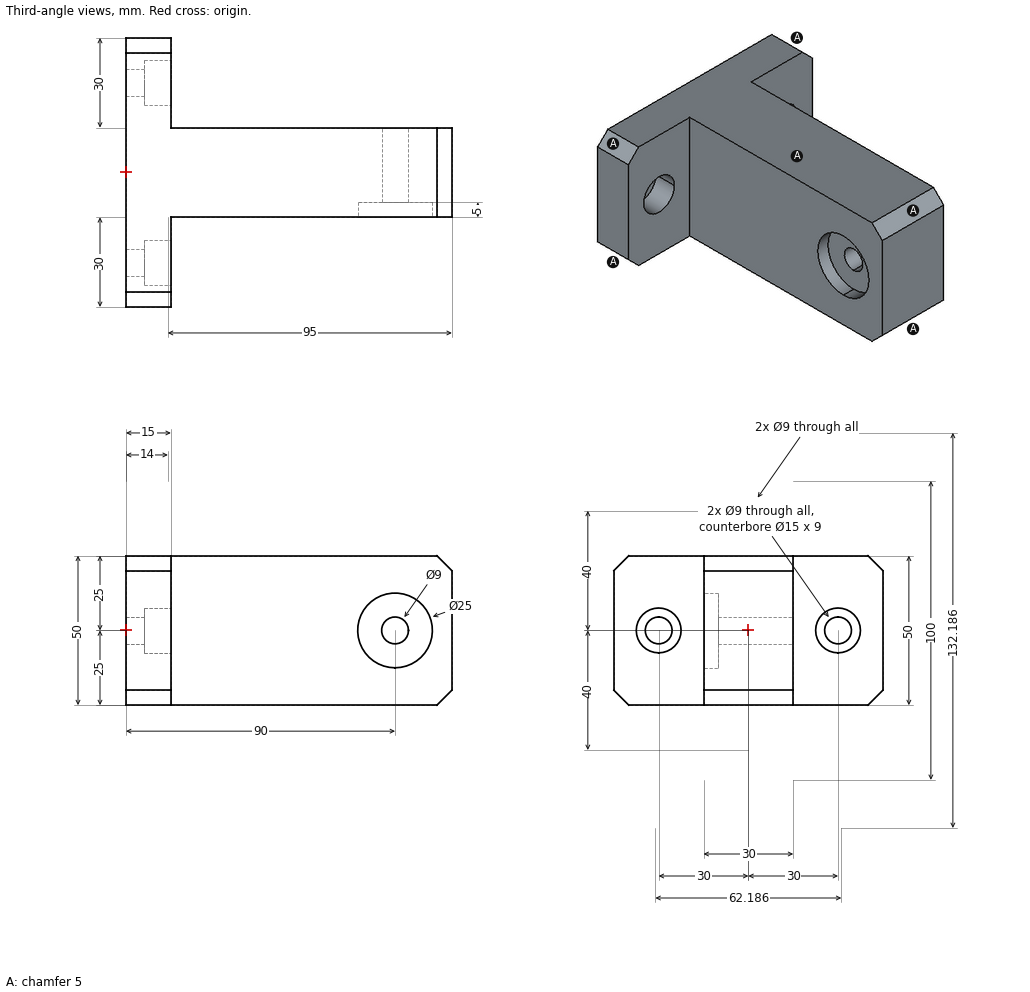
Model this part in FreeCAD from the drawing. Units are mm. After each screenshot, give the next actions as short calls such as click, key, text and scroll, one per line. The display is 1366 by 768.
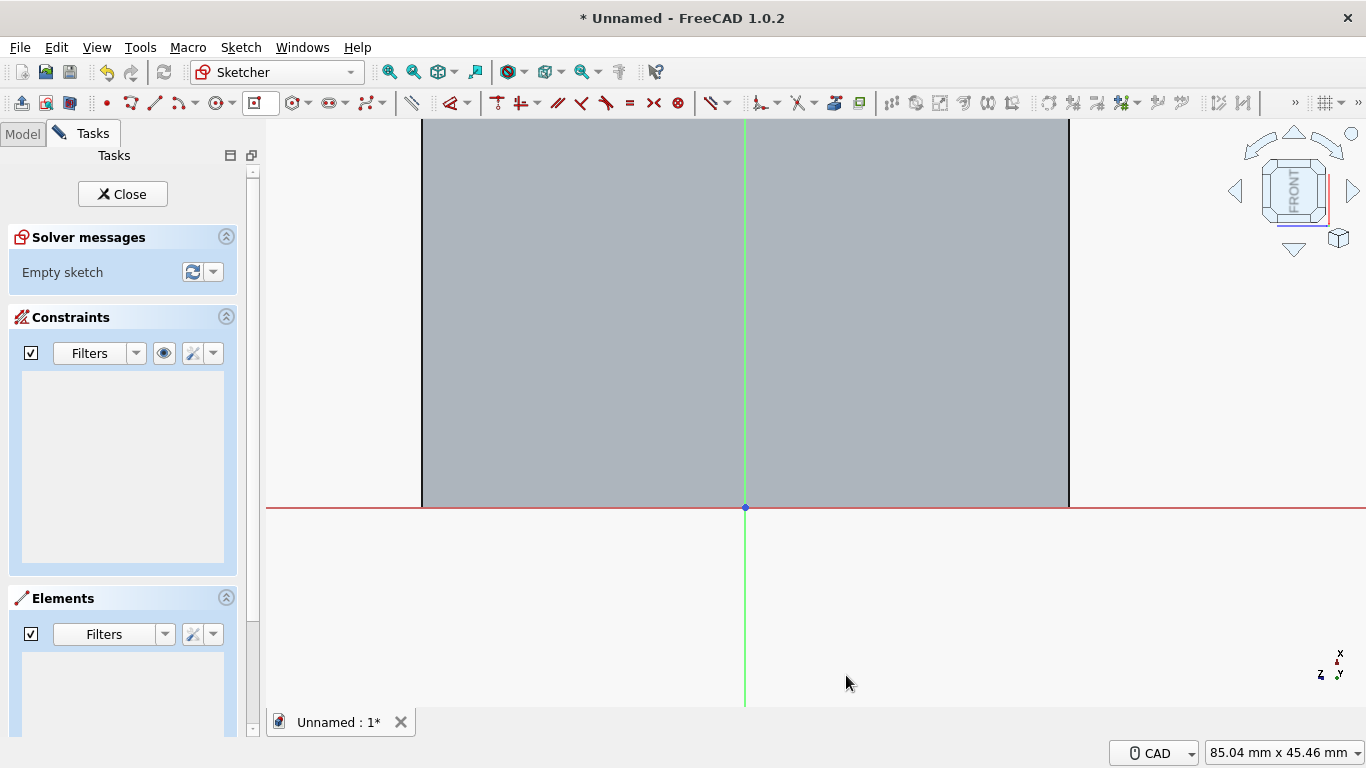
key(g)
key(r)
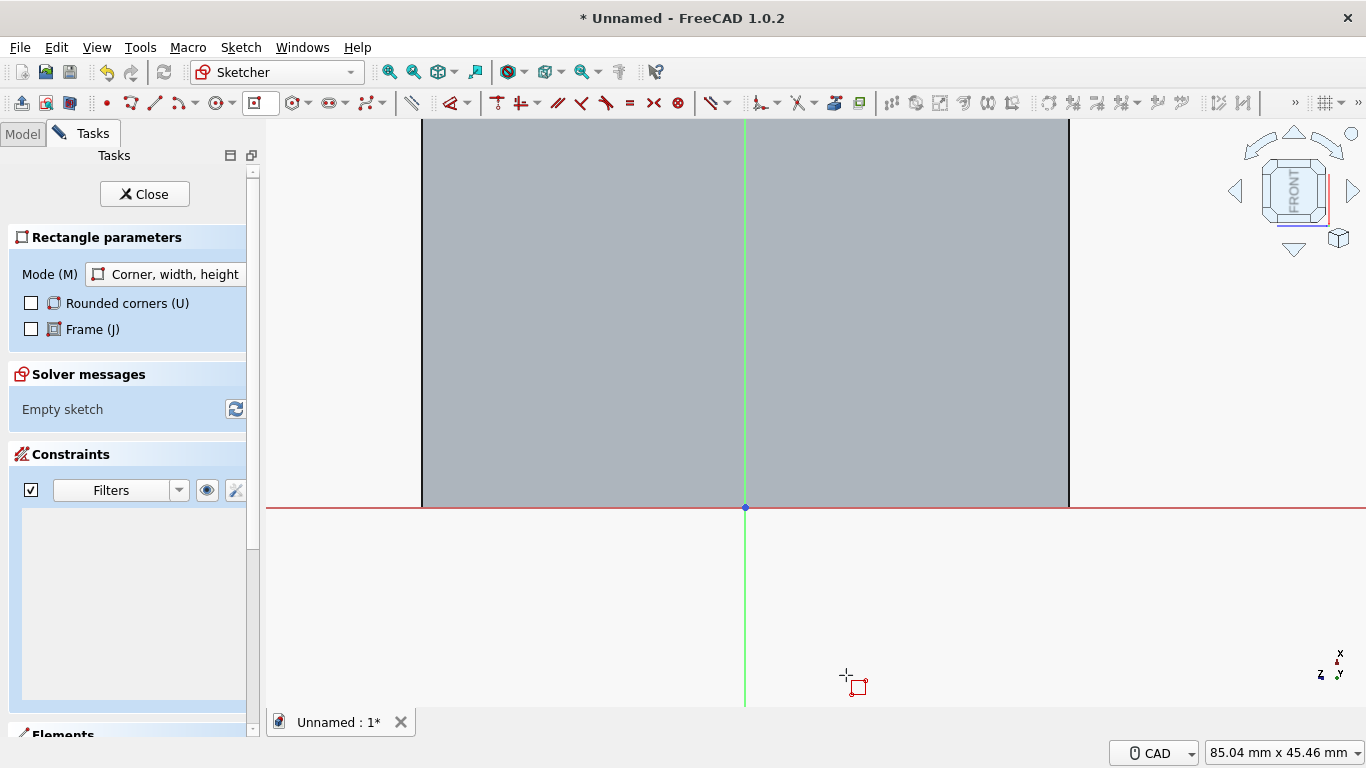
click(422, 314)
click(1069, 508)
key(Escape)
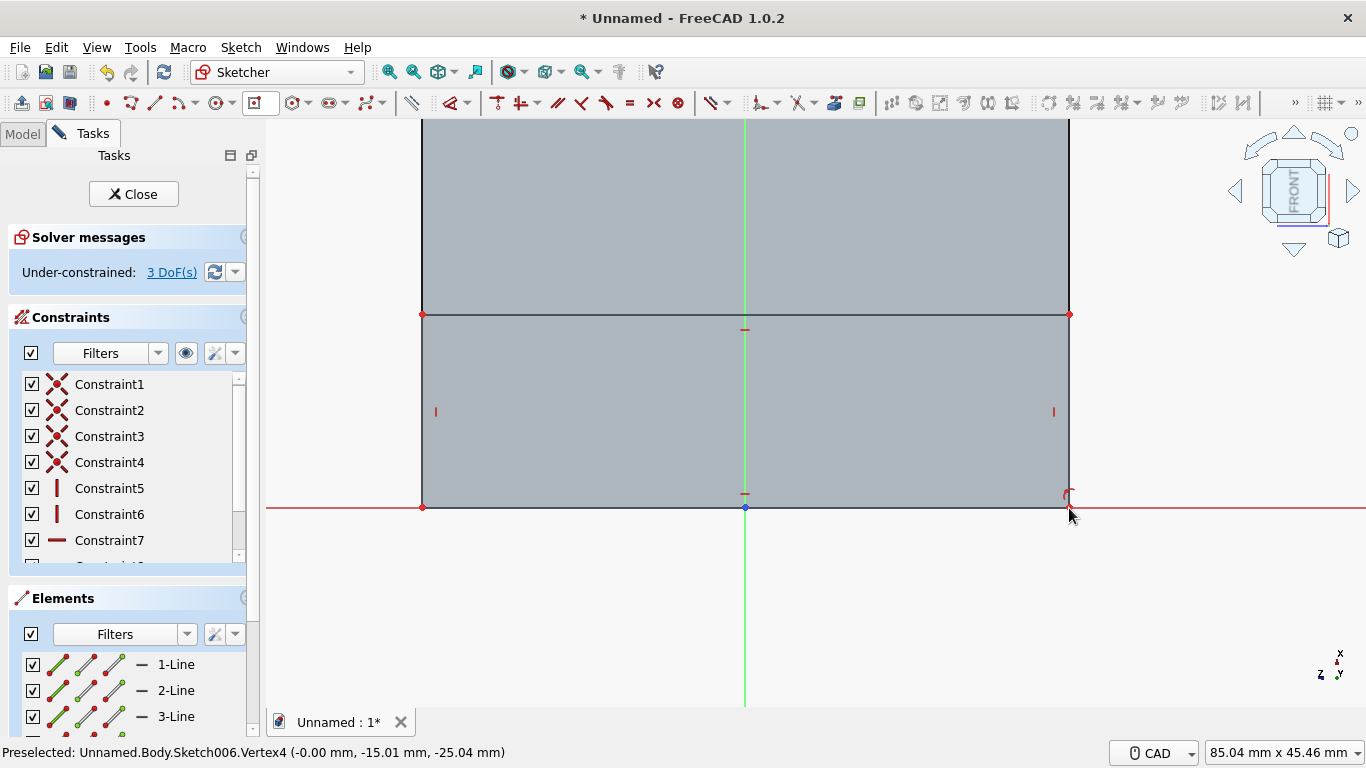
click(450, 104)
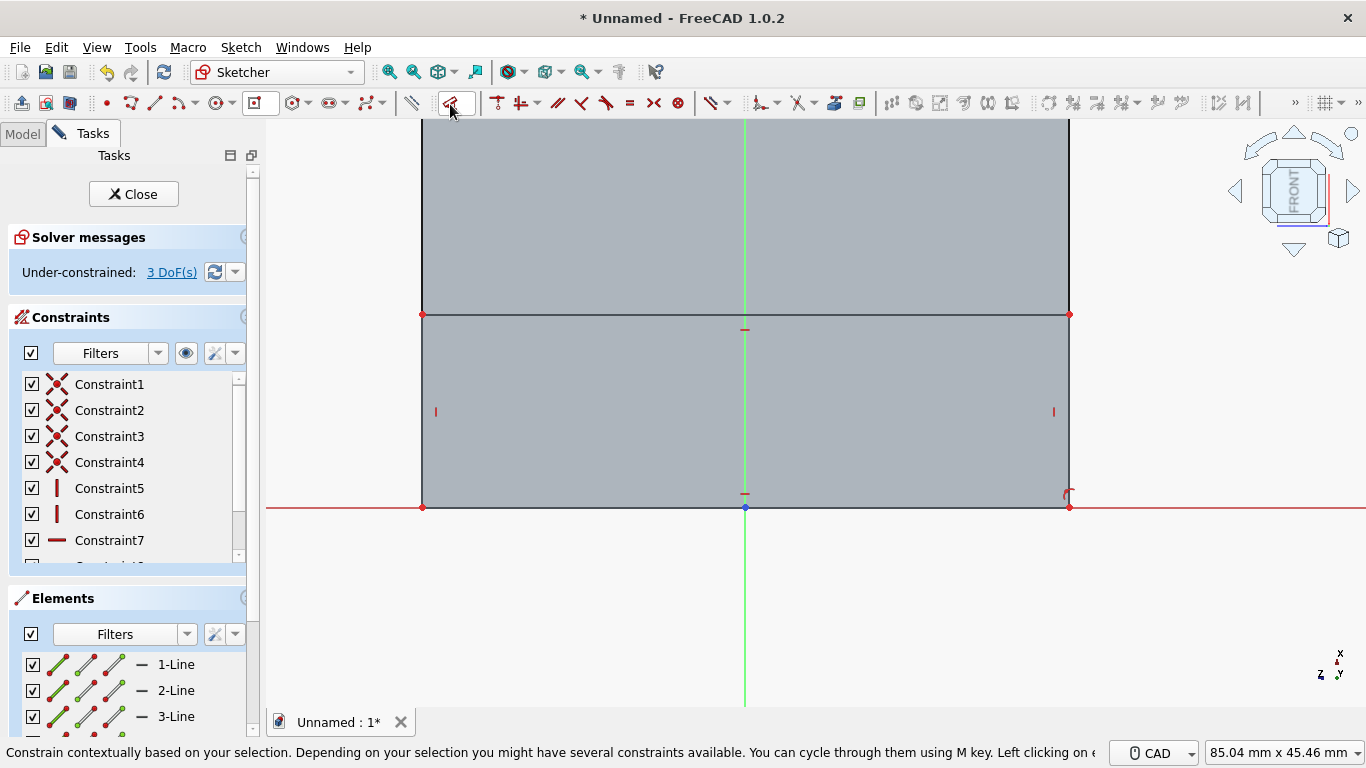
click(422, 373)
click(388, 411)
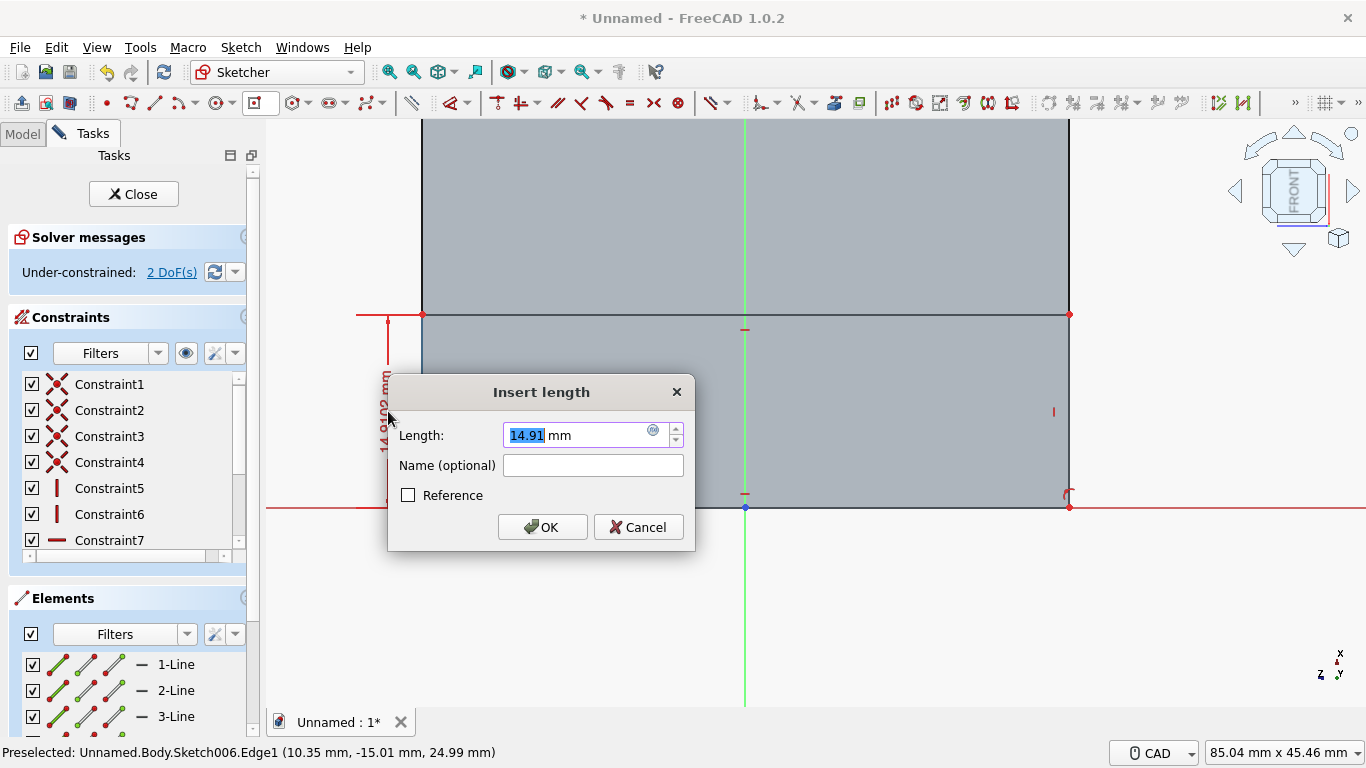
text(15)
key(Return)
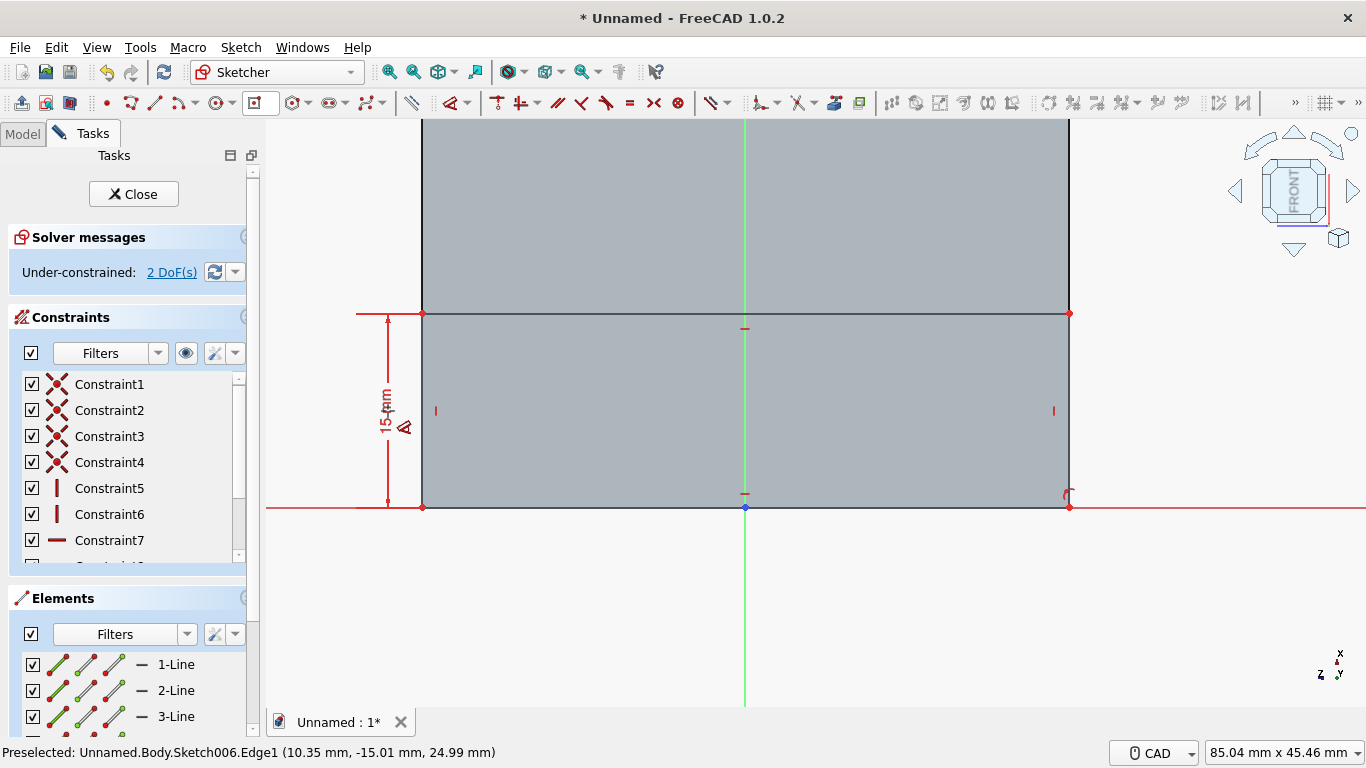
click(616, 508)
click(597, 542)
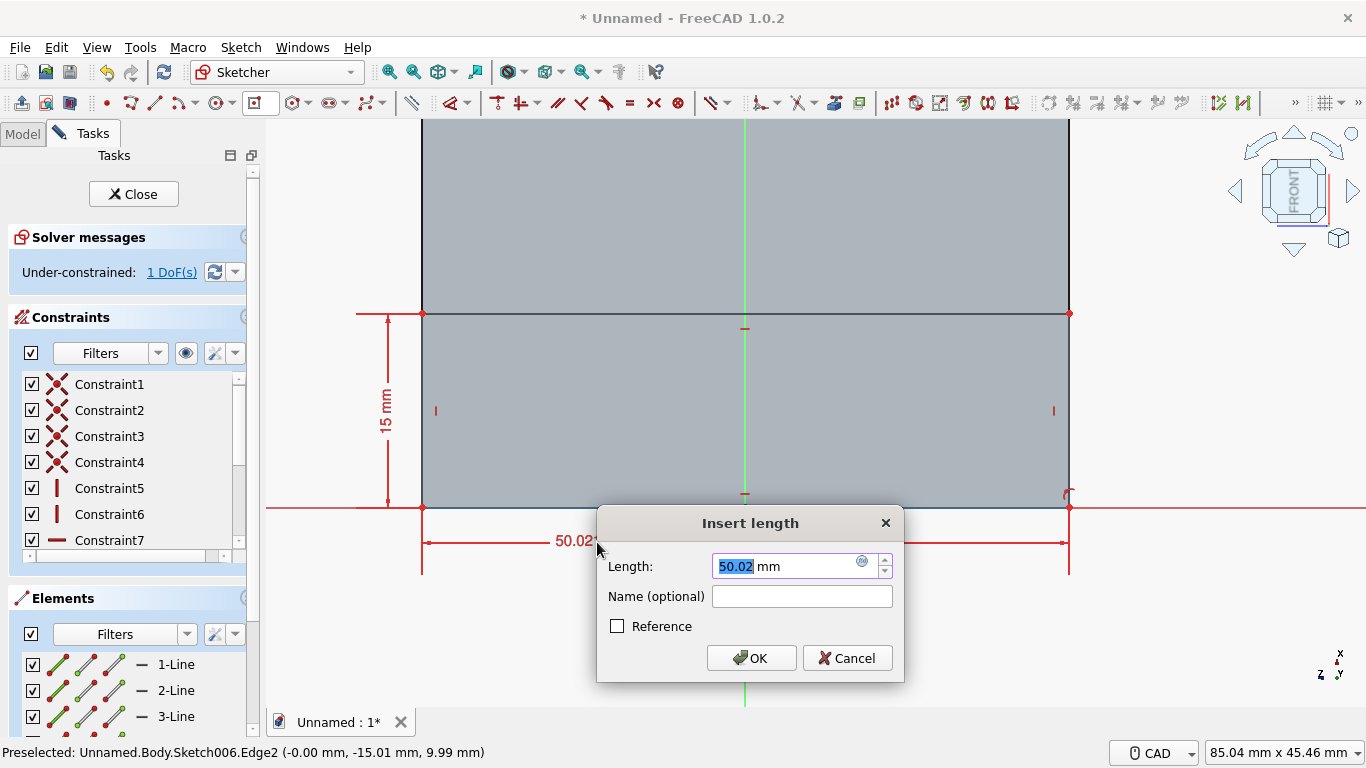
text(50)
key(Return)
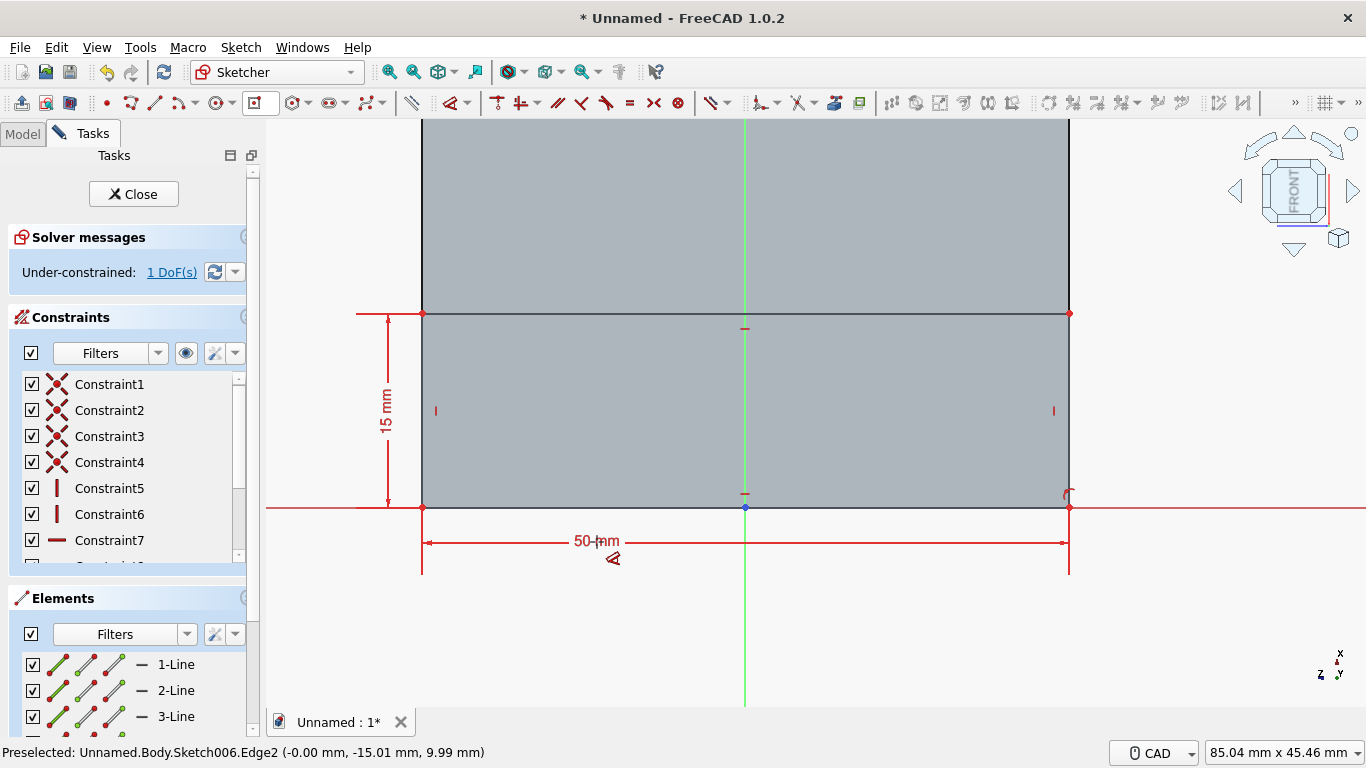
click(422, 314)
click(509, 542)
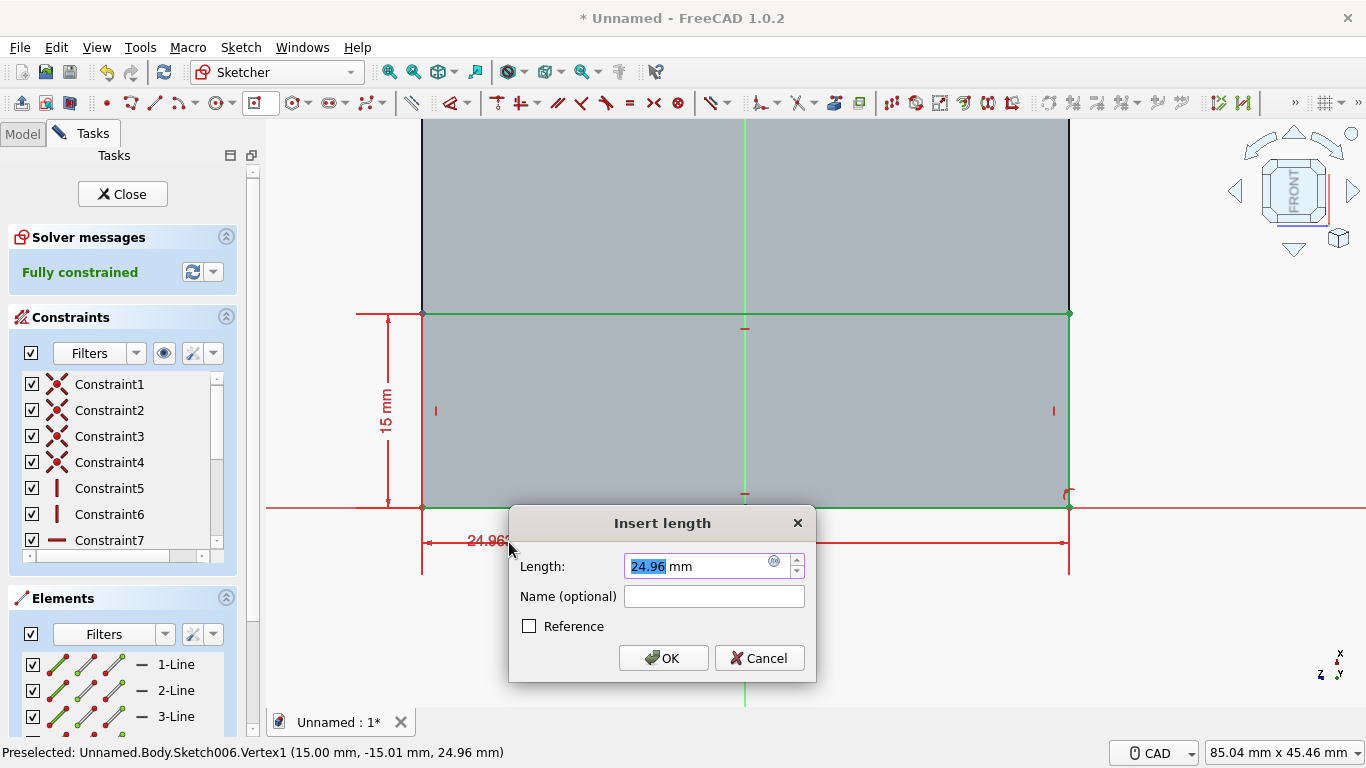
text(25)
key(Return)
key(Escape)